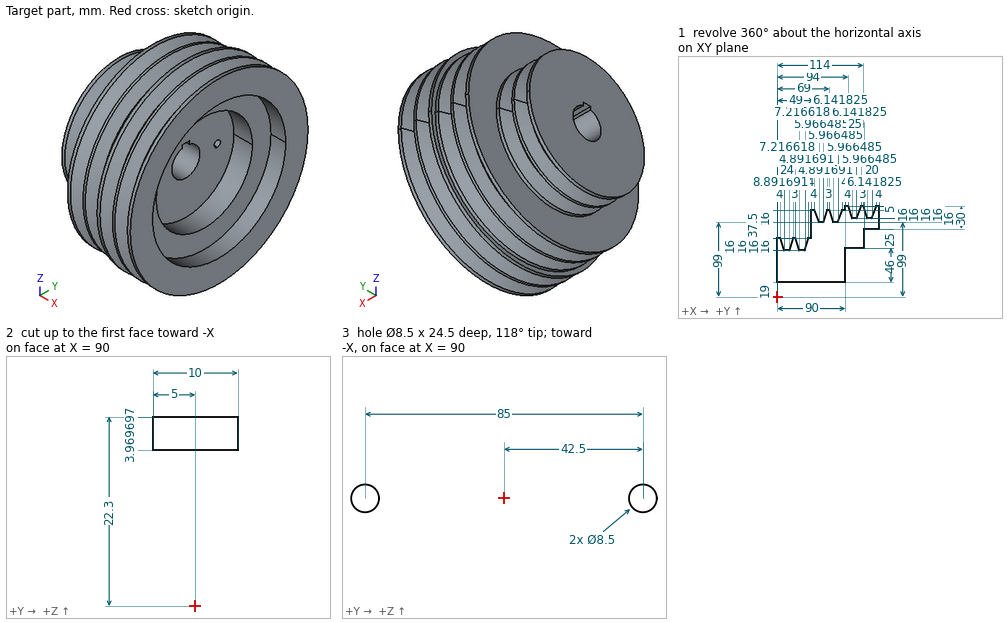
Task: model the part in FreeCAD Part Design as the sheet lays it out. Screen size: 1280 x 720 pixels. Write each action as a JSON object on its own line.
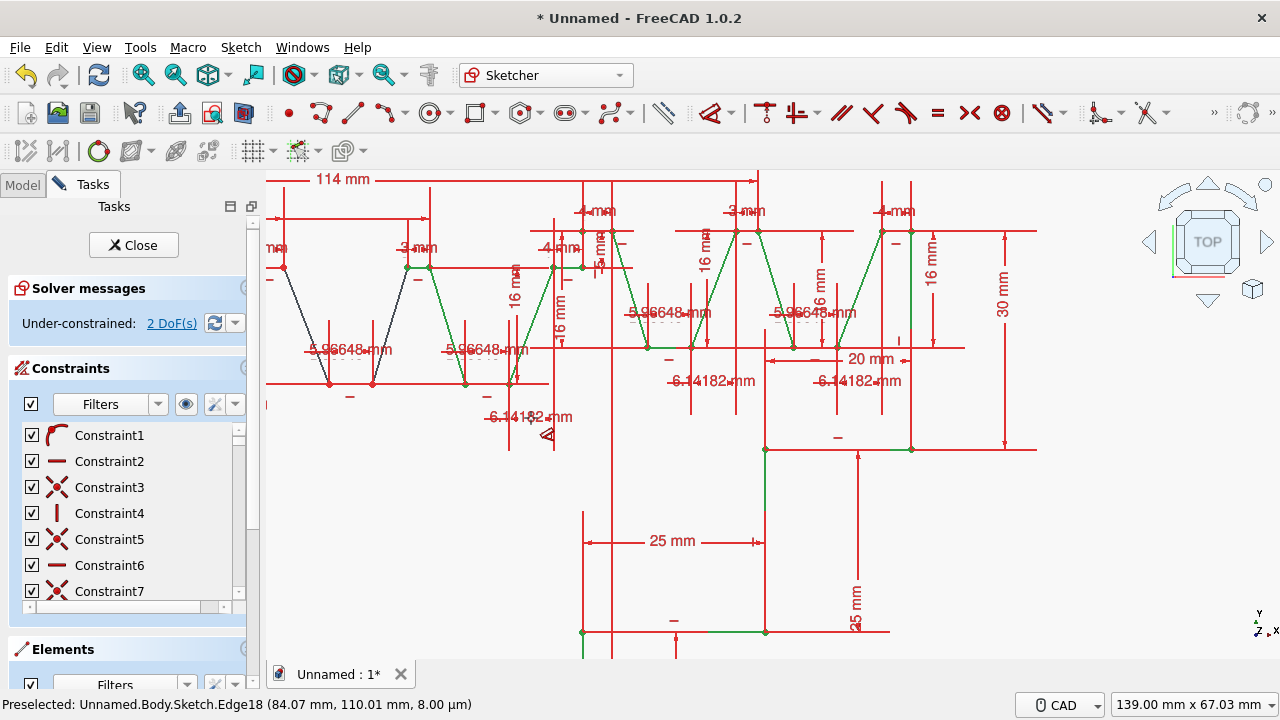
{"action": "left_click", "coordinate": [397, 303]}
{"action": "left_click", "coordinate": [390, 418]}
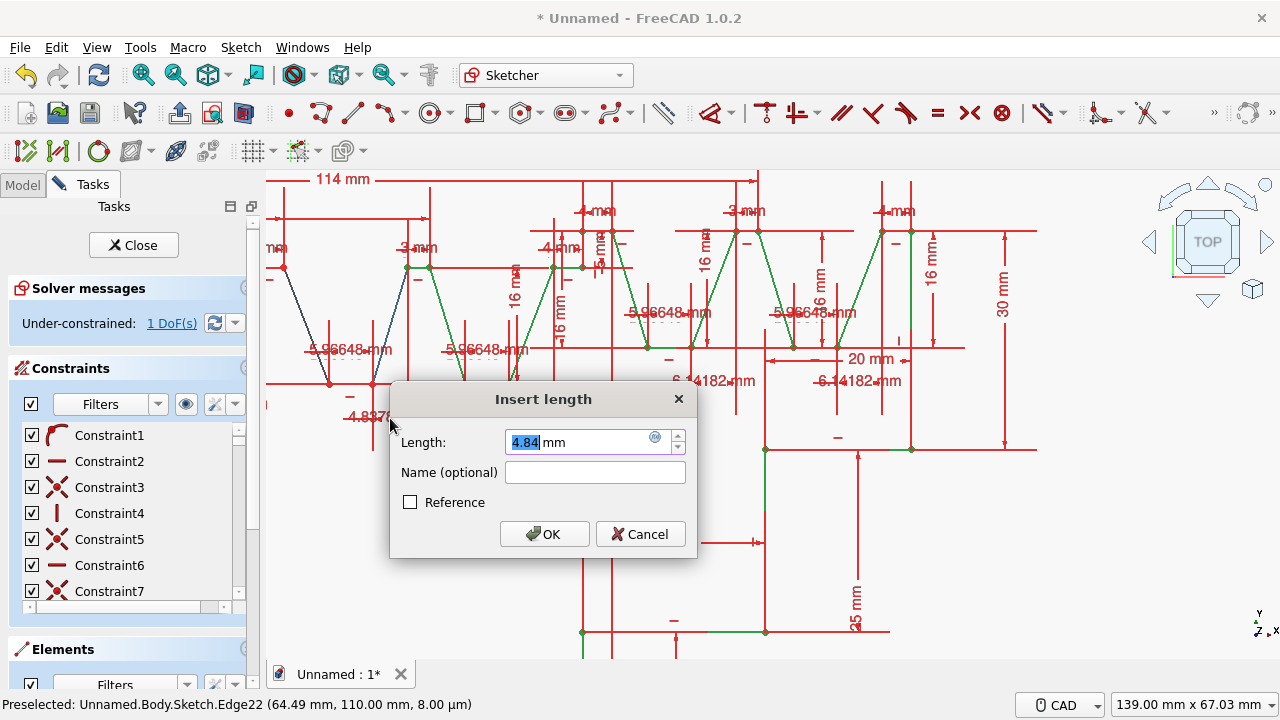
{"action": "type", "text": "4.891691"}
{"action": "key", "text": "Return"}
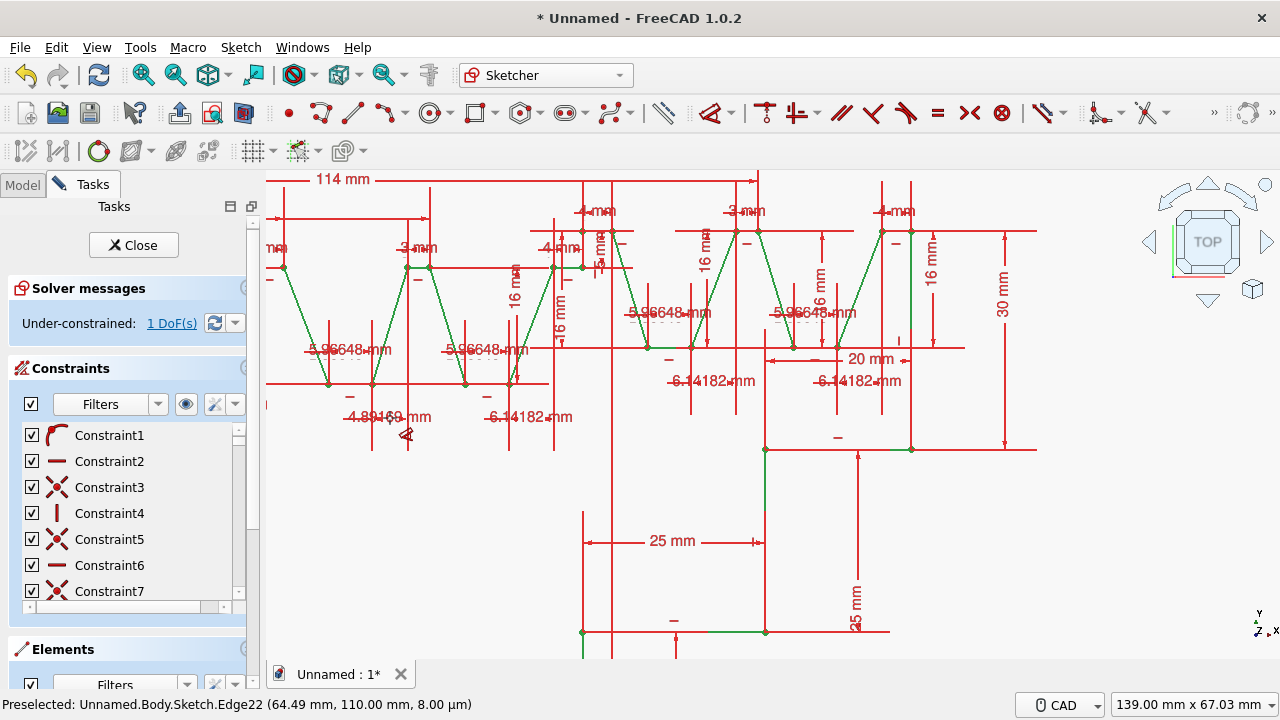
{"action": "scroll", "coordinate": [871, 267], "scroll_direction": "down", "scroll_amount": 5}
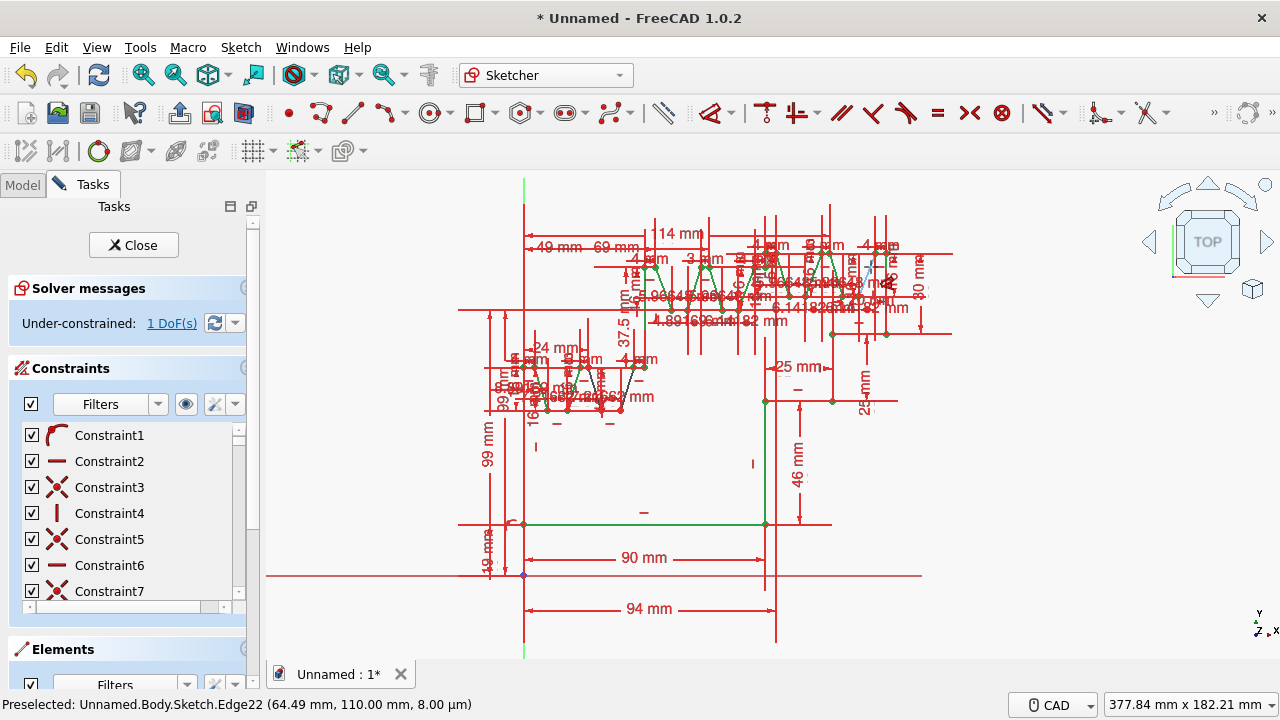
{"action": "scroll", "coordinate": [630, 381], "scroll_direction": "up", "scroll_amount": 6}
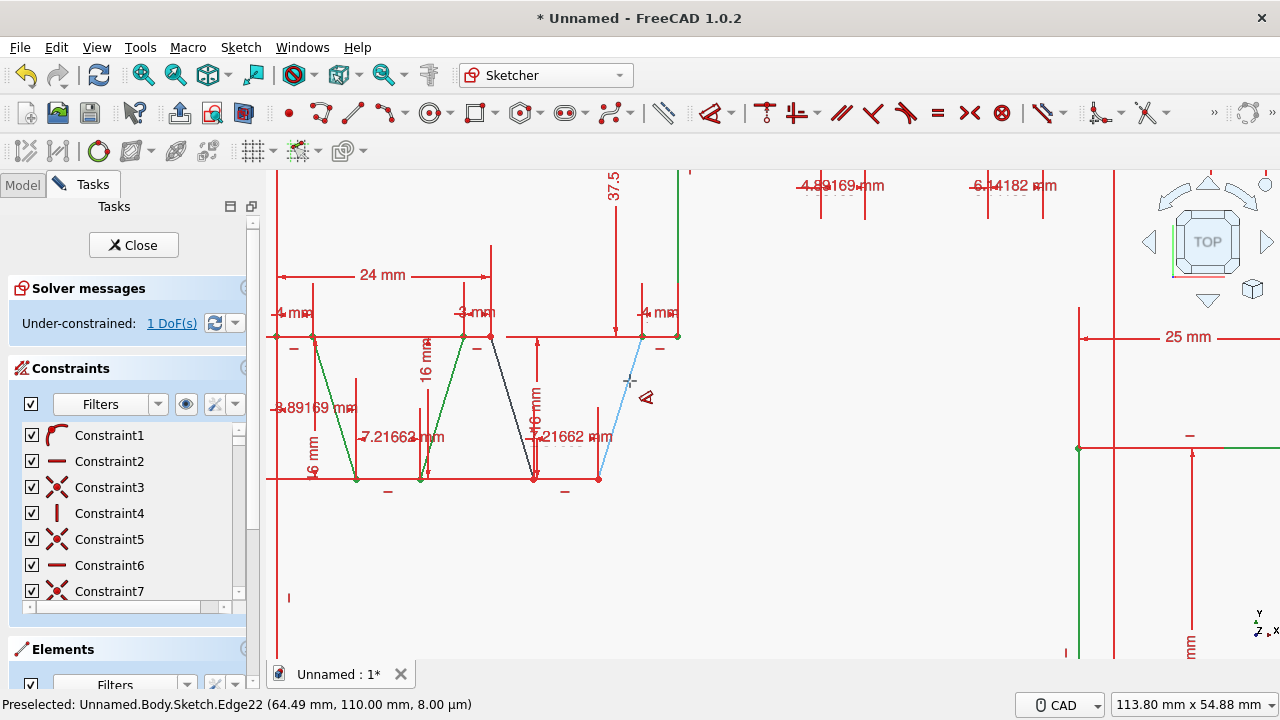
{"action": "left_click", "coordinate": [629, 379]}
{"action": "left_click", "coordinate": [620, 513]}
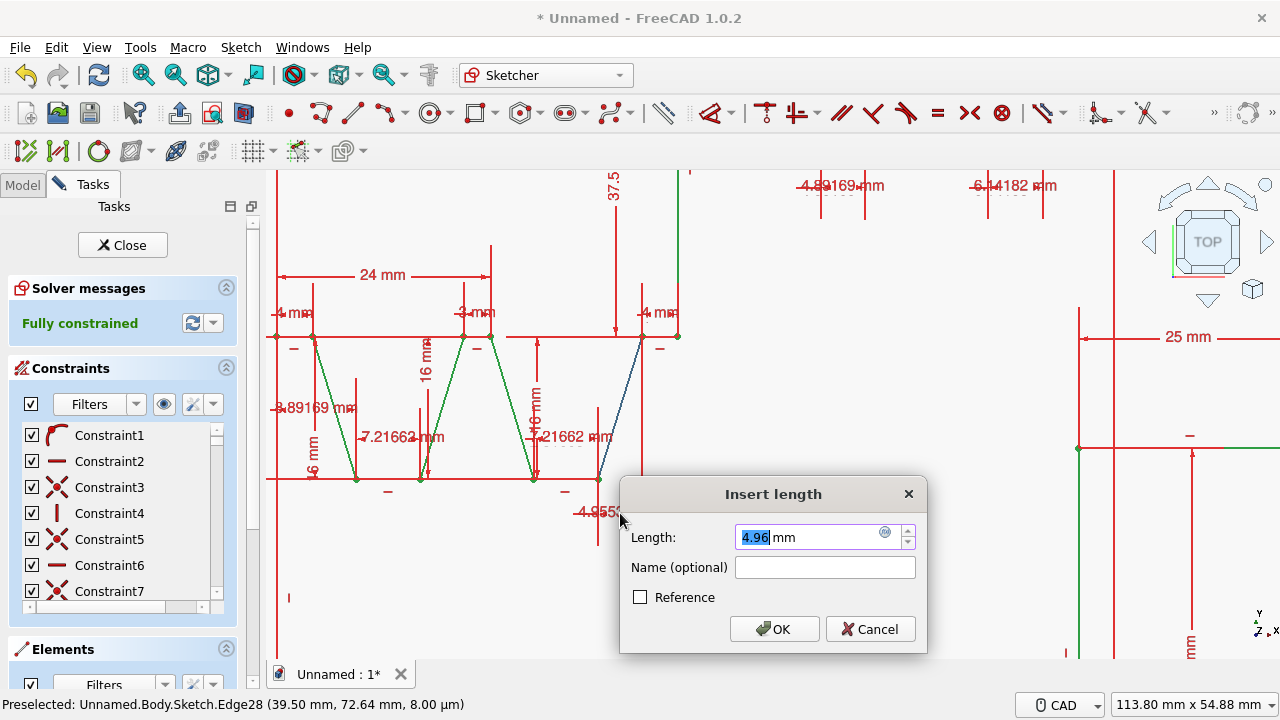
{"action": "type", "text": "4.891691"}
{"action": "key", "text": "Return"}
{"action": "key", "text": "Escape"}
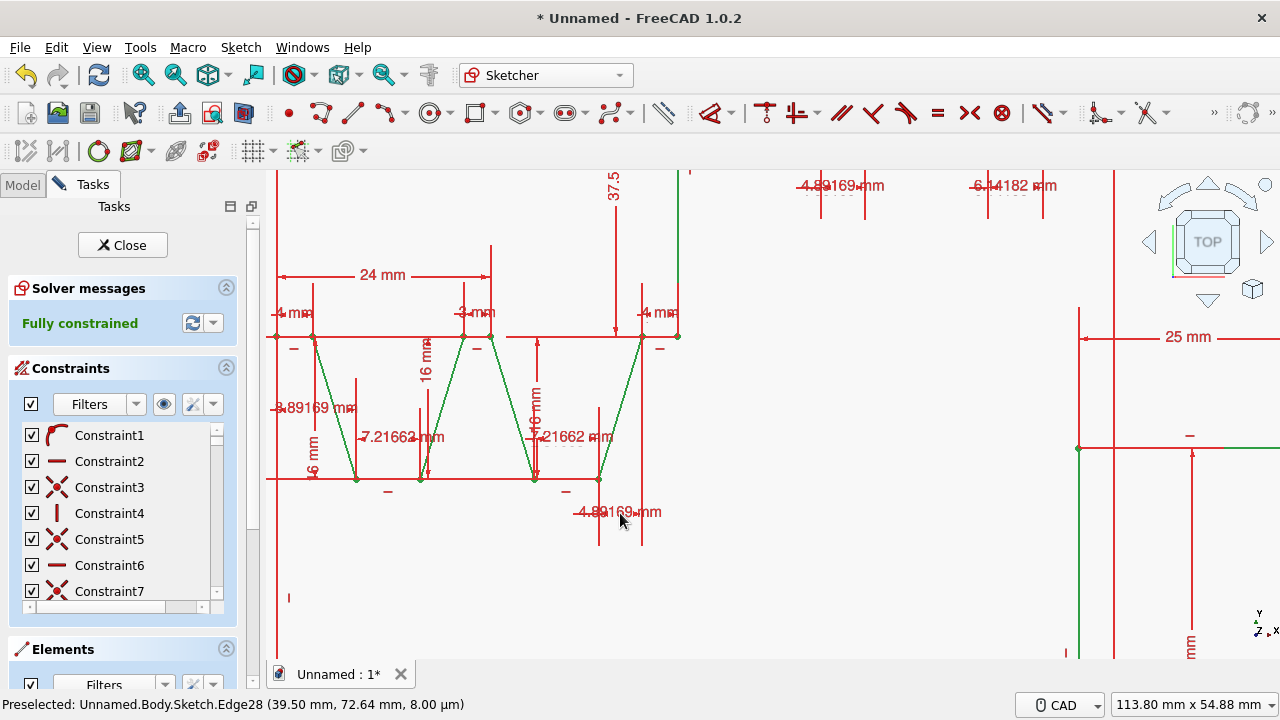
{"action": "left_click", "coordinate": [123, 245]}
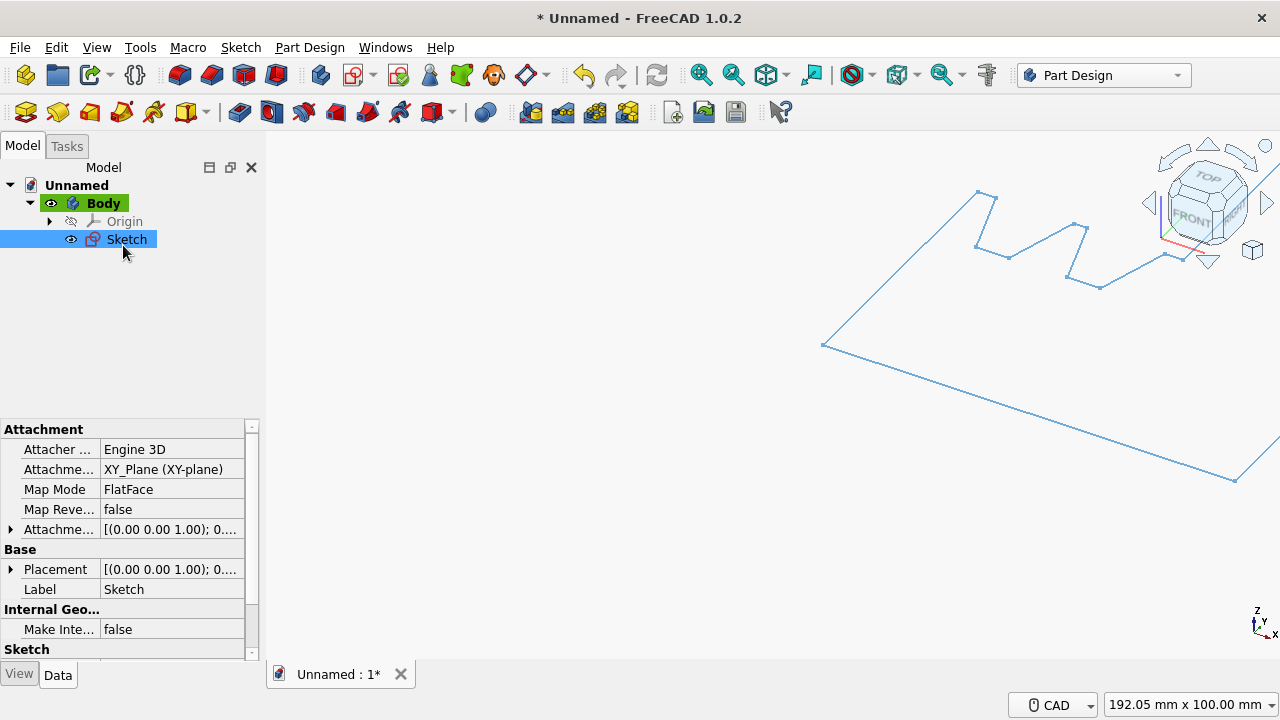
{"action": "left_click", "coordinate": [58, 112]}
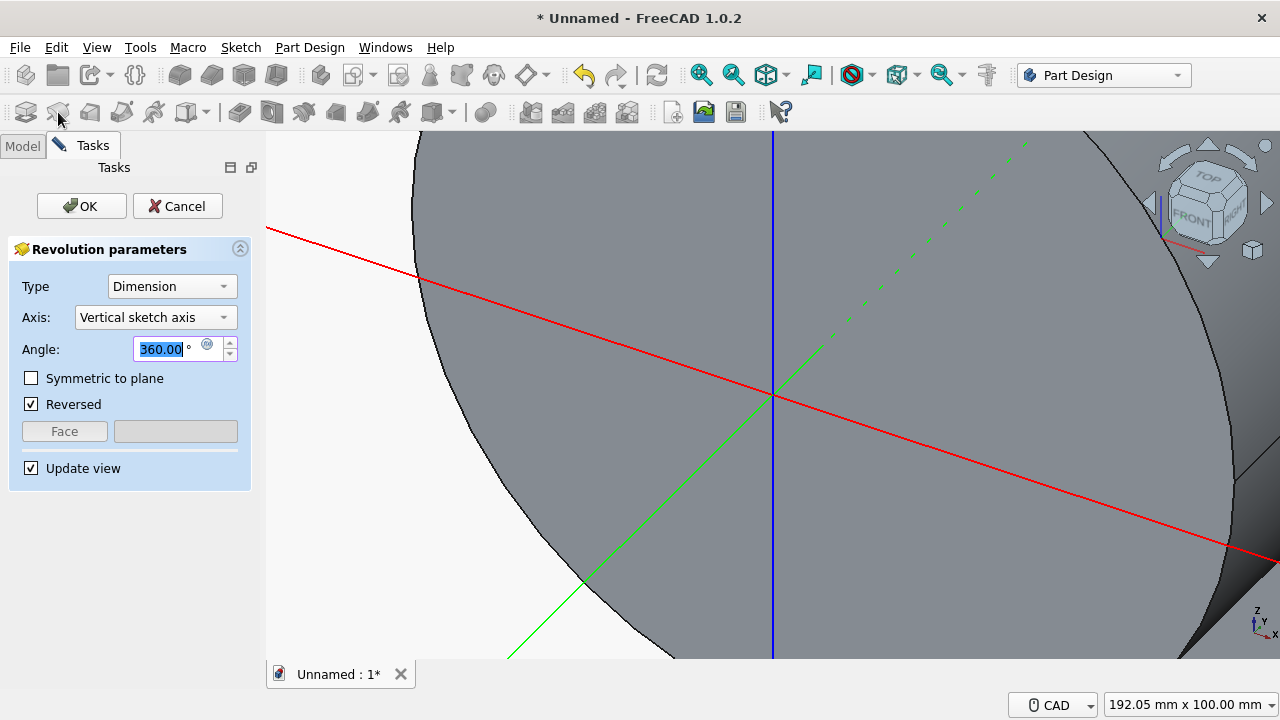
{"action": "left_click", "coordinate": [156, 318]}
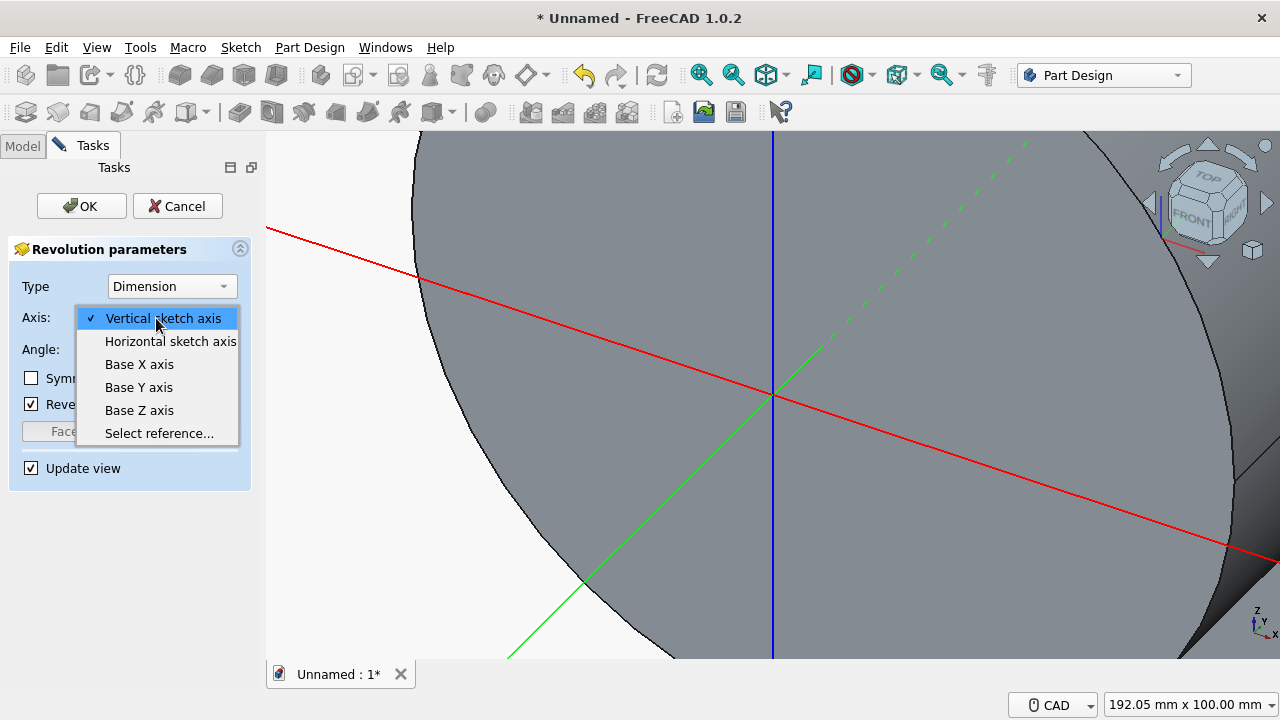
{"action": "left_click", "coordinate": [156, 342]}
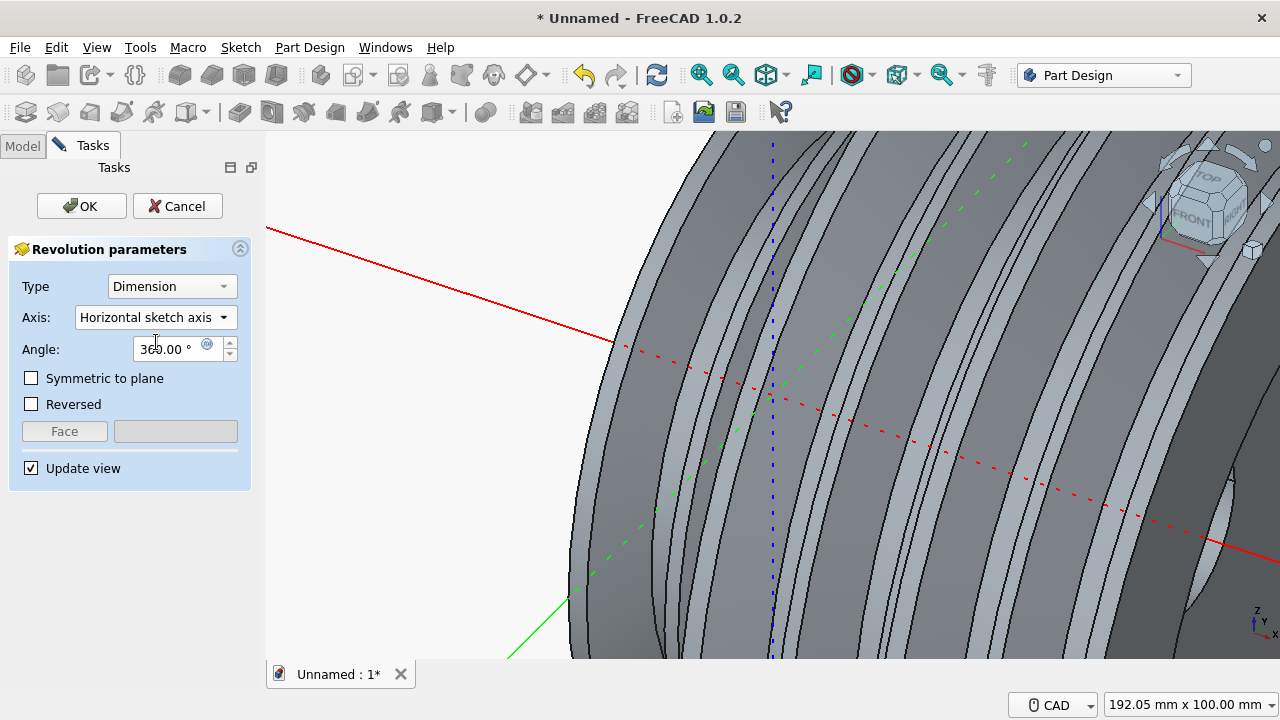
{"action": "left_click", "coordinate": [82, 206]}